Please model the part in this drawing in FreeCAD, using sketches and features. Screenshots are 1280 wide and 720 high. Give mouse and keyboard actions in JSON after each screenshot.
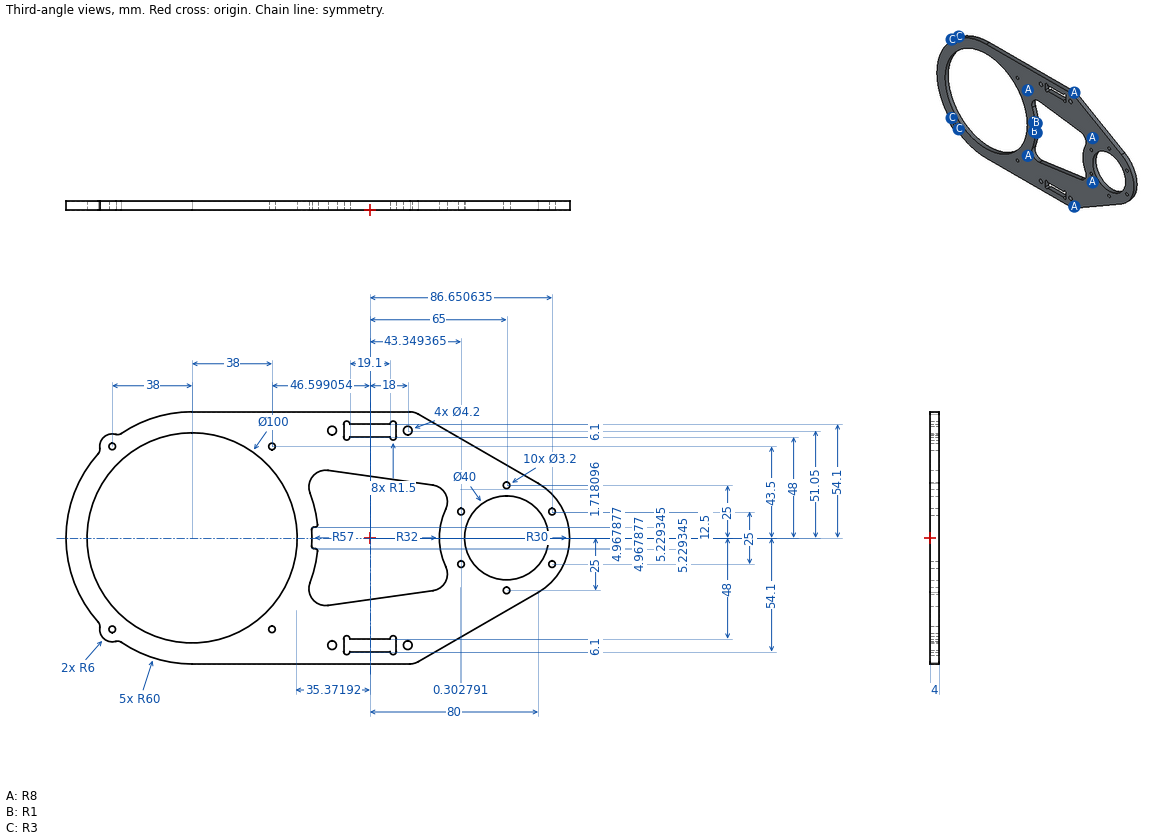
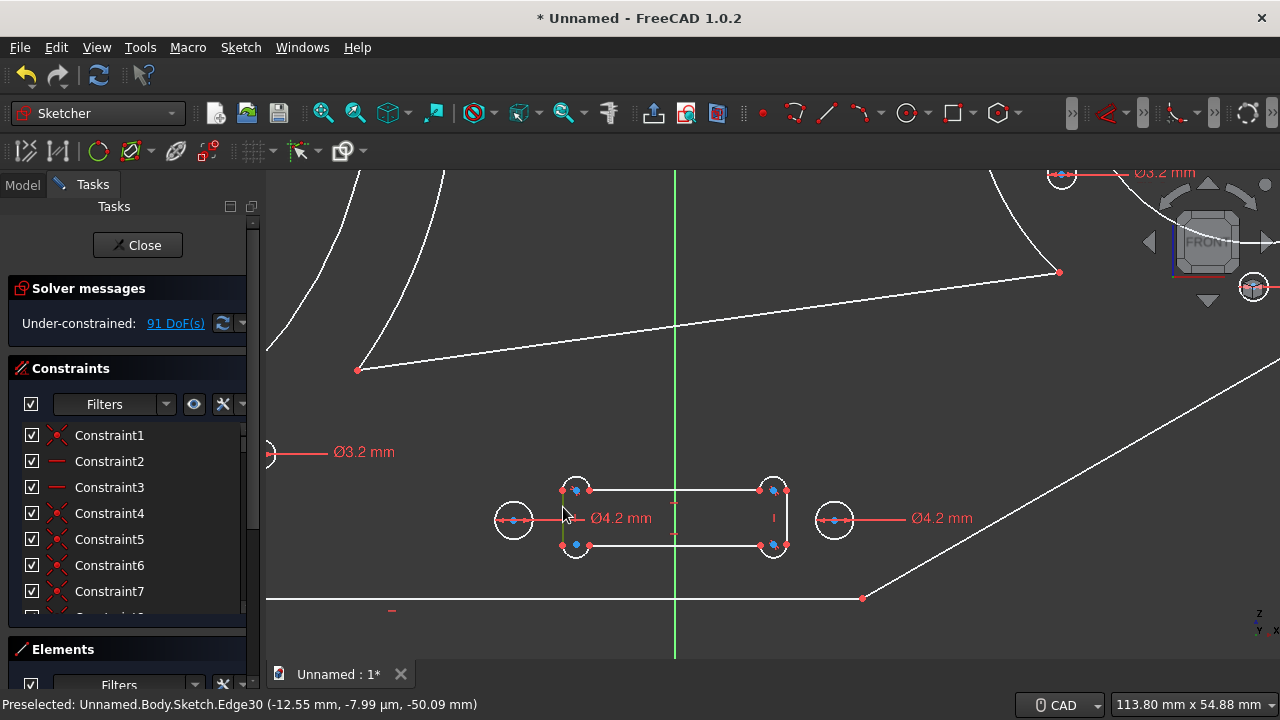
{"action": "left_click", "coordinate": [568, 555]}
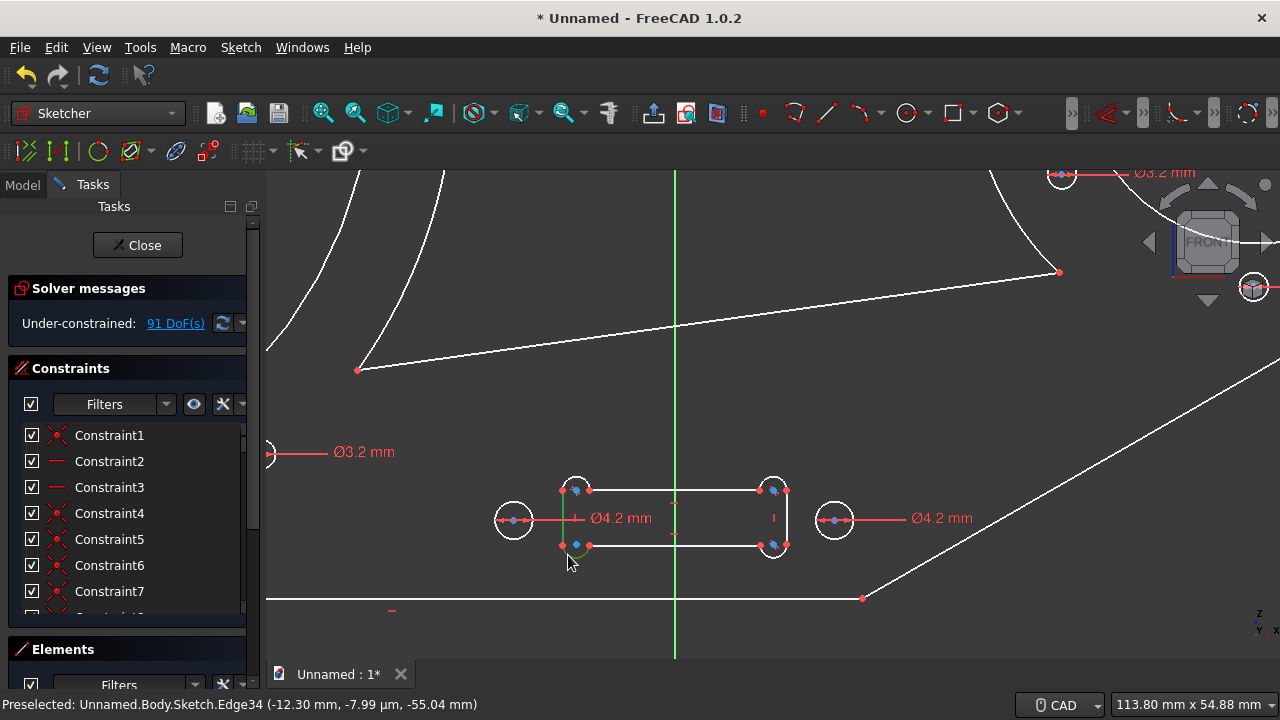
{"action": "key", "text": "t"}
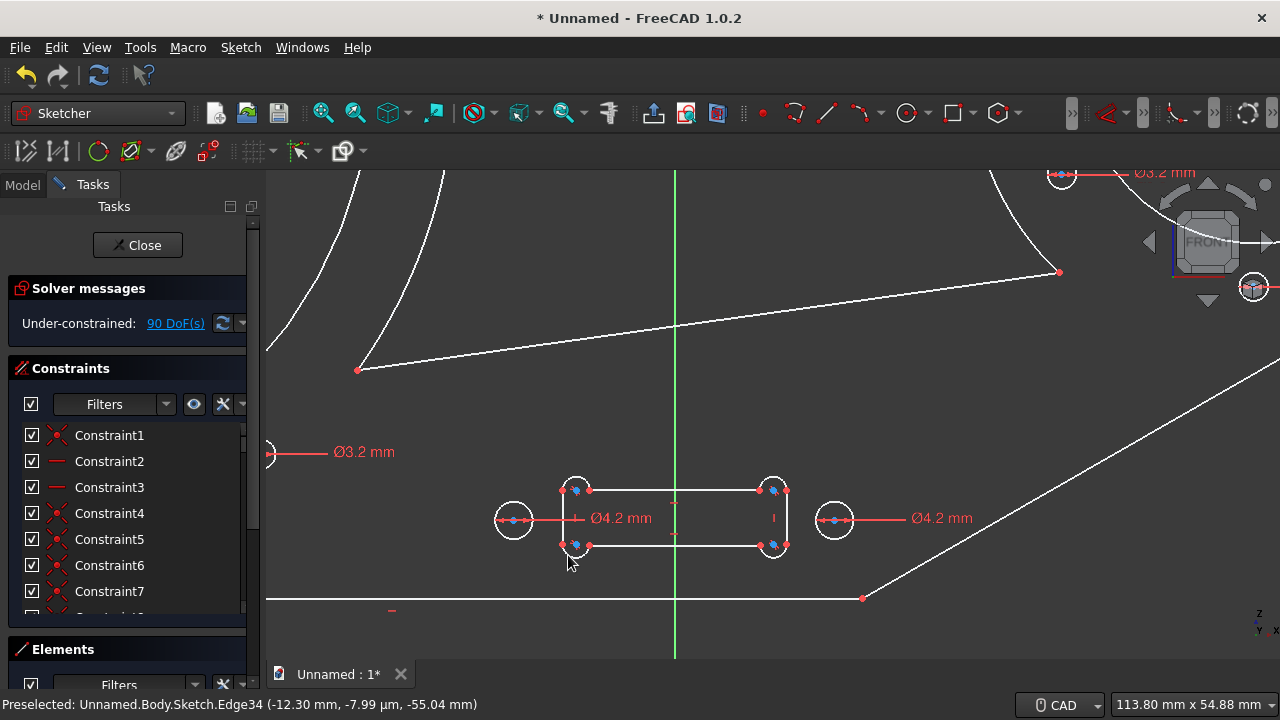
{"action": "scroll", "coordinate": [787, 530], "scroll_direction": "down", "scroll_amount": 7}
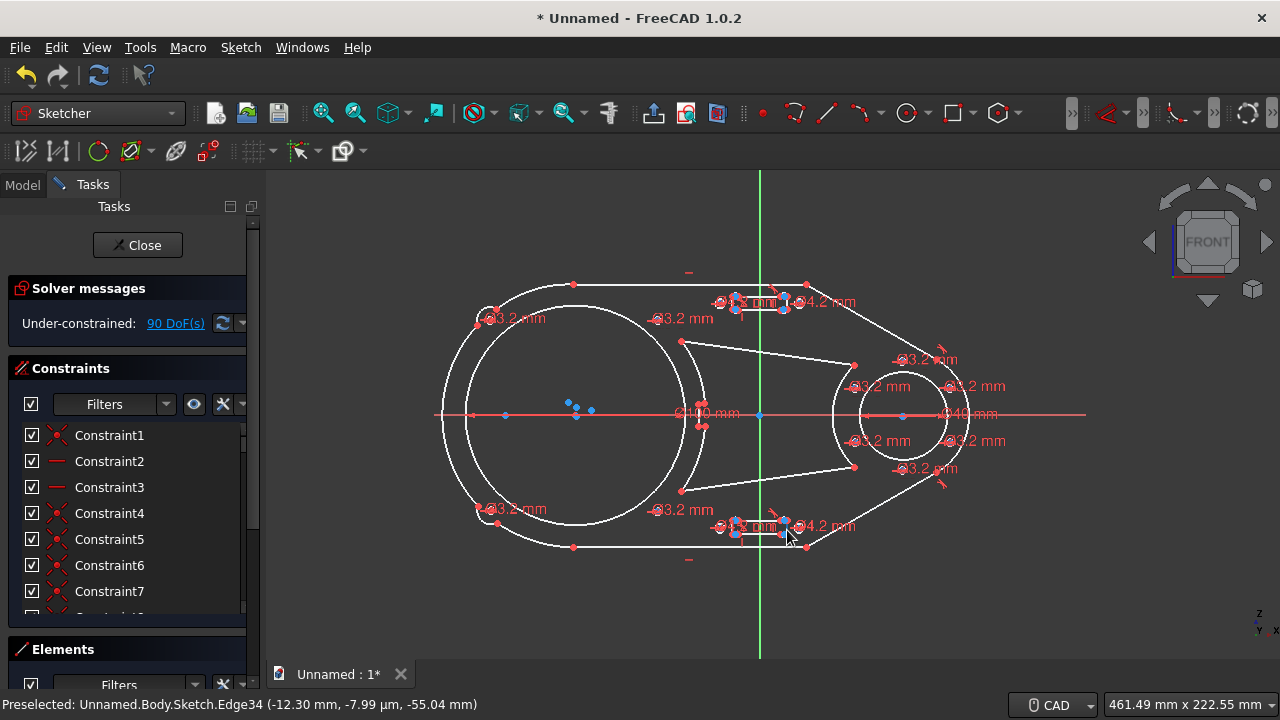
{"action": "left_click", "coordinate": [653, 337]}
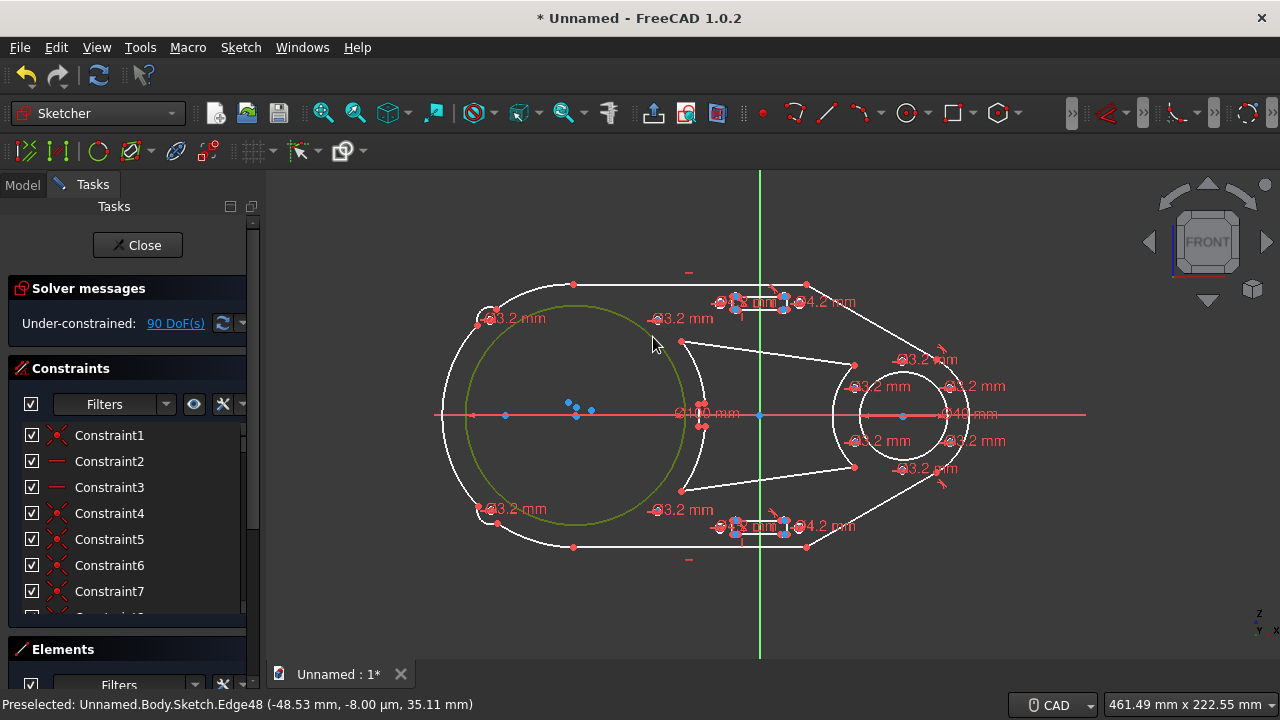
{"action": "left_click", "coordinate": [518, 535]}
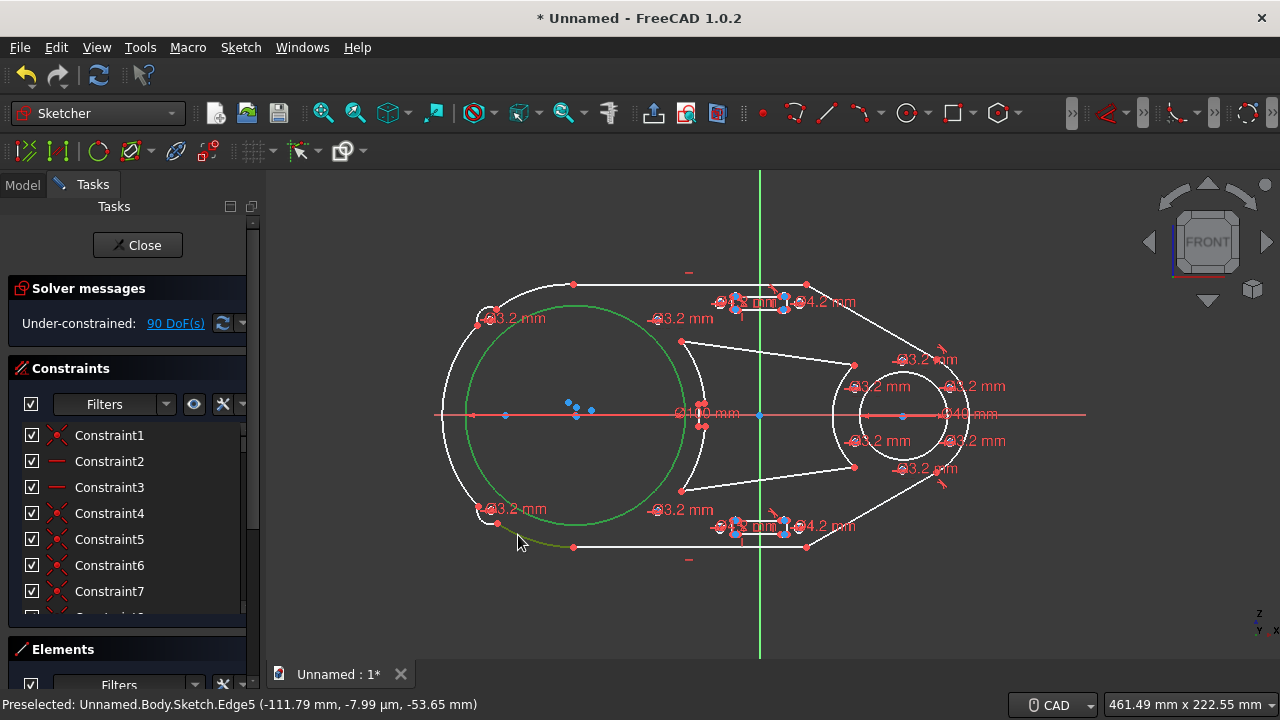
{"action": "key", "text": "c"}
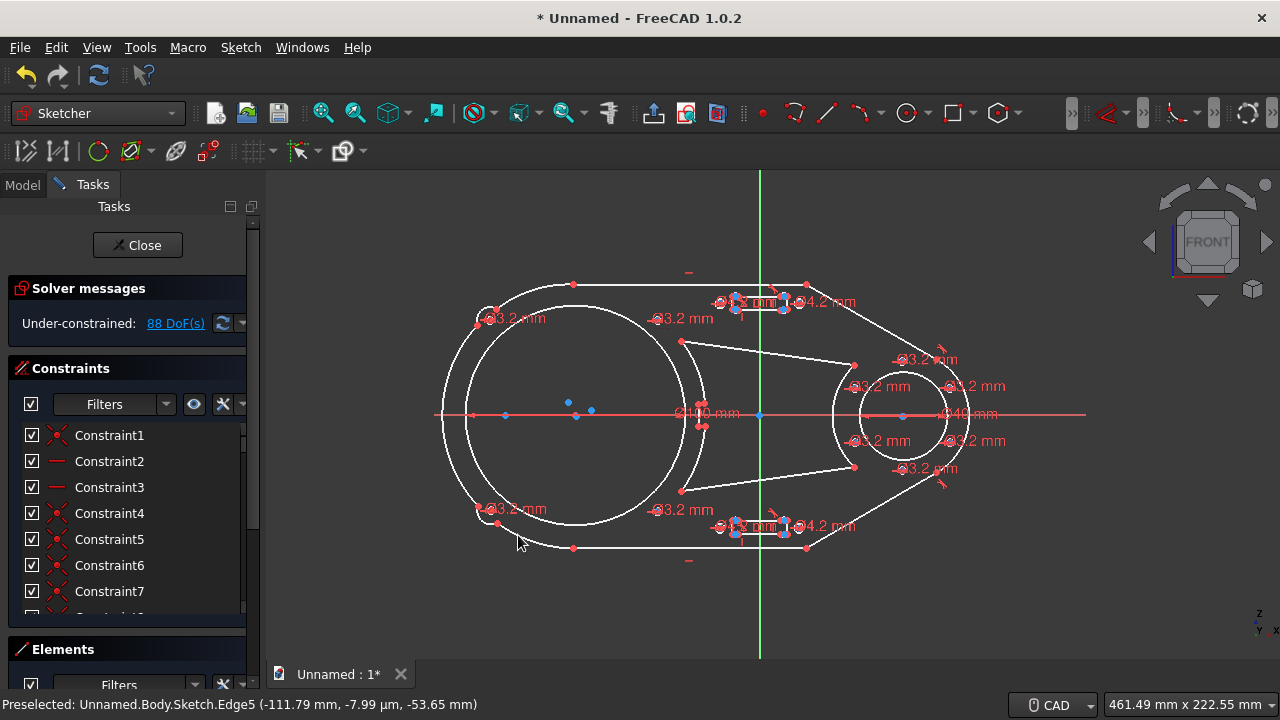
{"action": "left_click", "coordinate": [653, 337]}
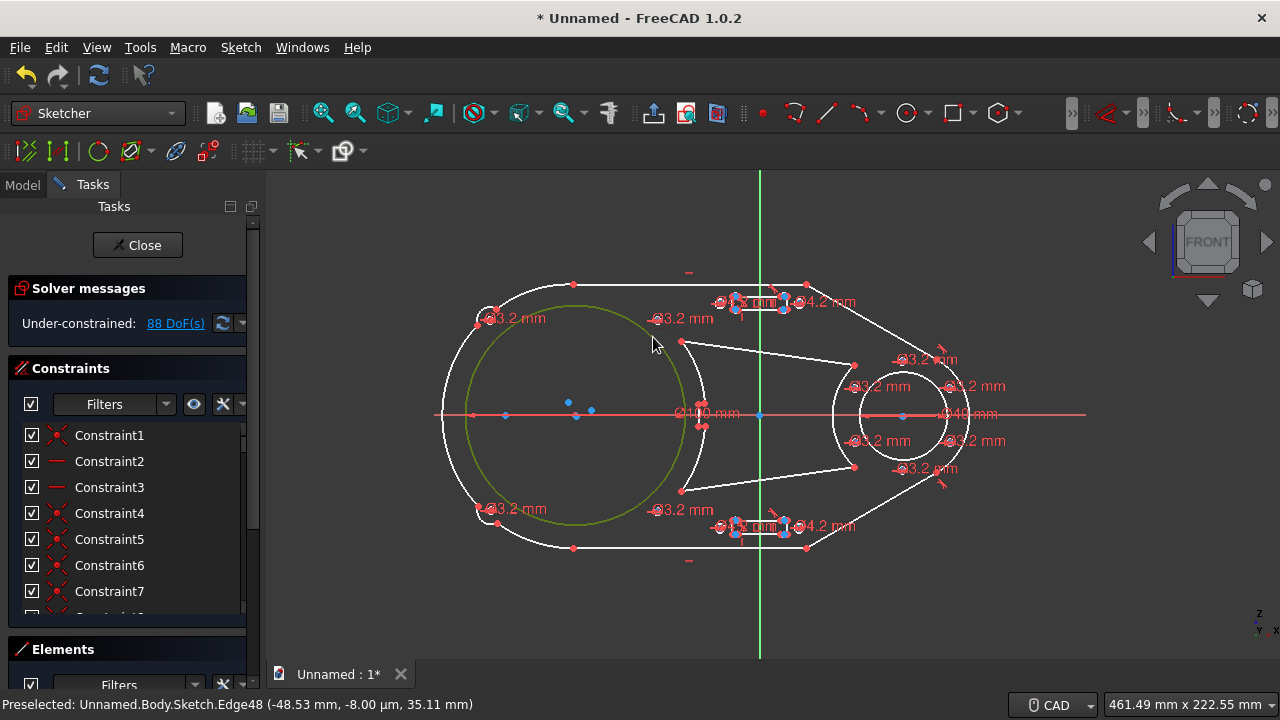
{"action": "left_click", "coordinate": [549, 286]}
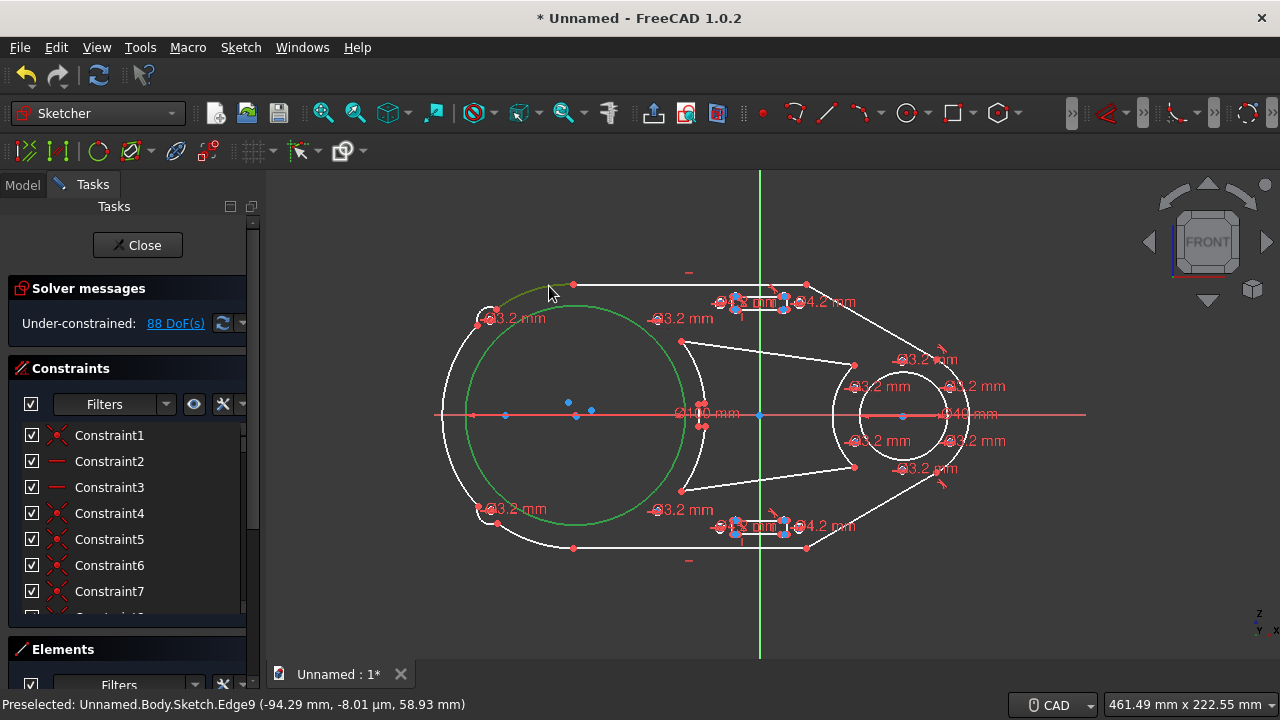
{"action": "key", "text": "c"}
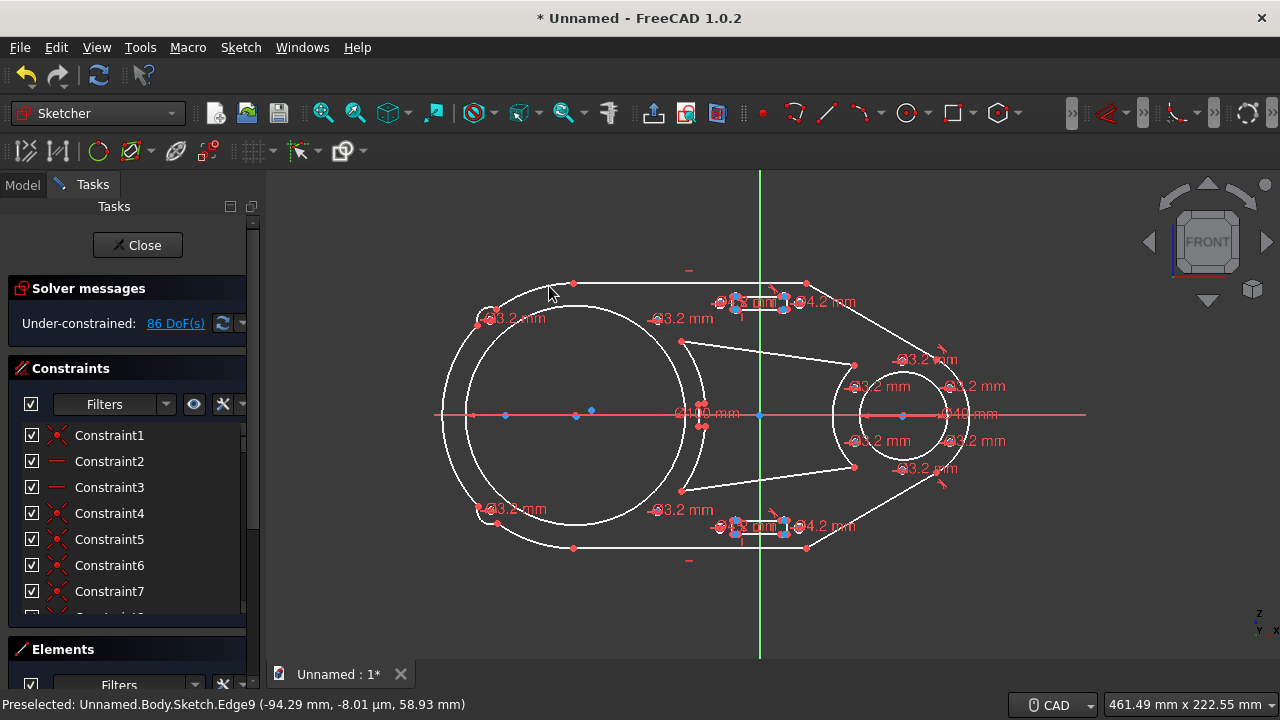
{"action": "left_click", "coordinate": [935, 385]}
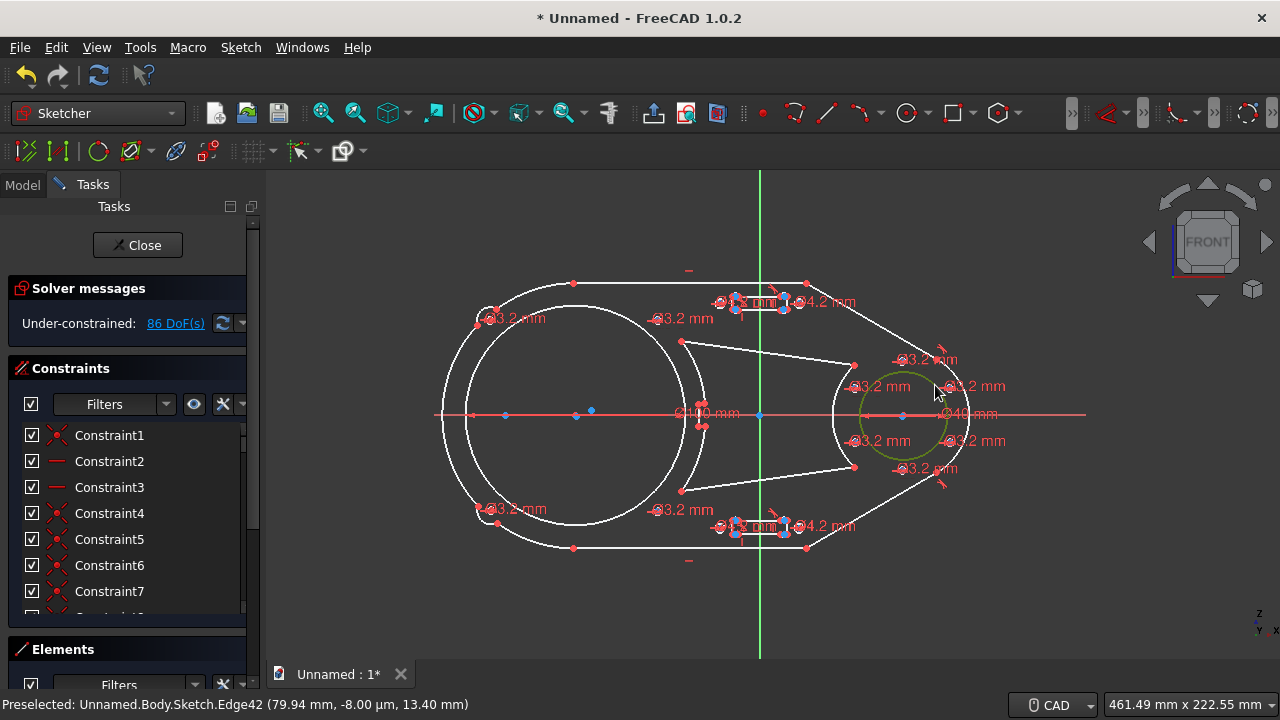
{"action": "left_click", "coordinate": [836, 394]}